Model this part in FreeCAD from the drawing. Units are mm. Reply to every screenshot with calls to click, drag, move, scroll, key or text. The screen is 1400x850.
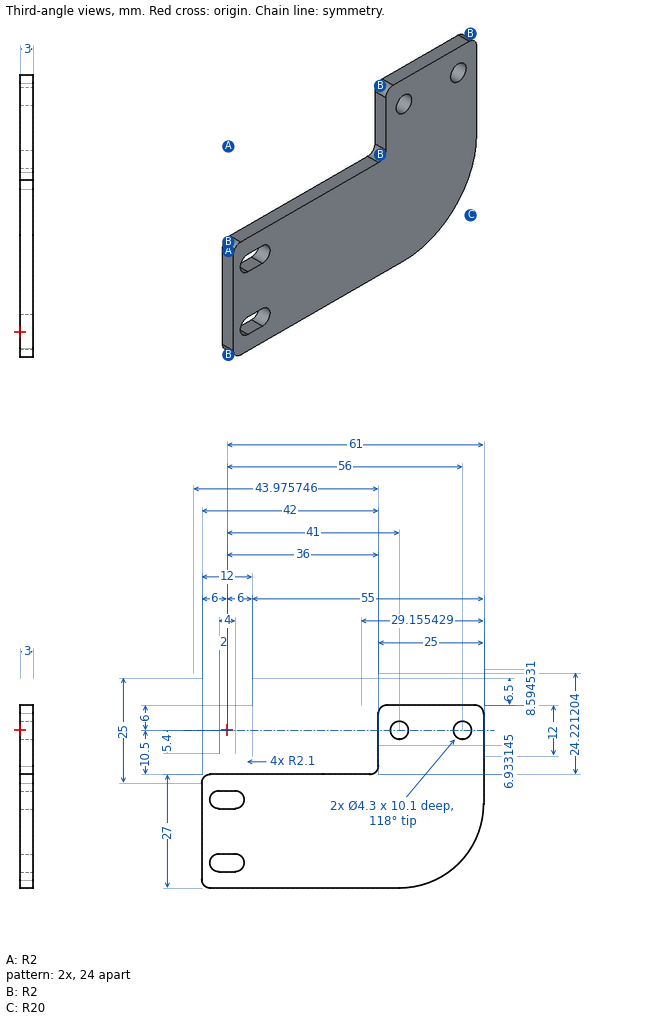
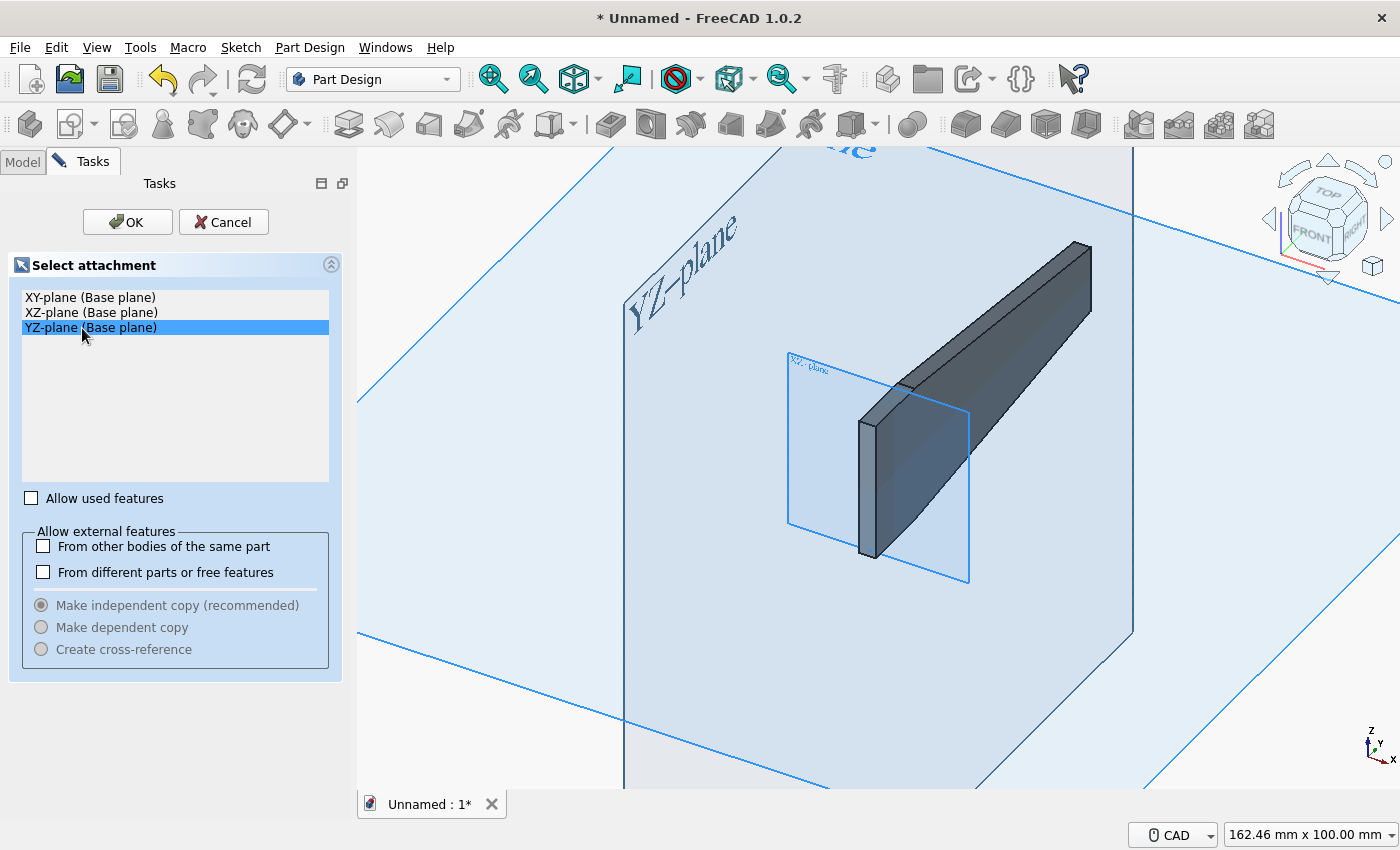
click(128, 222)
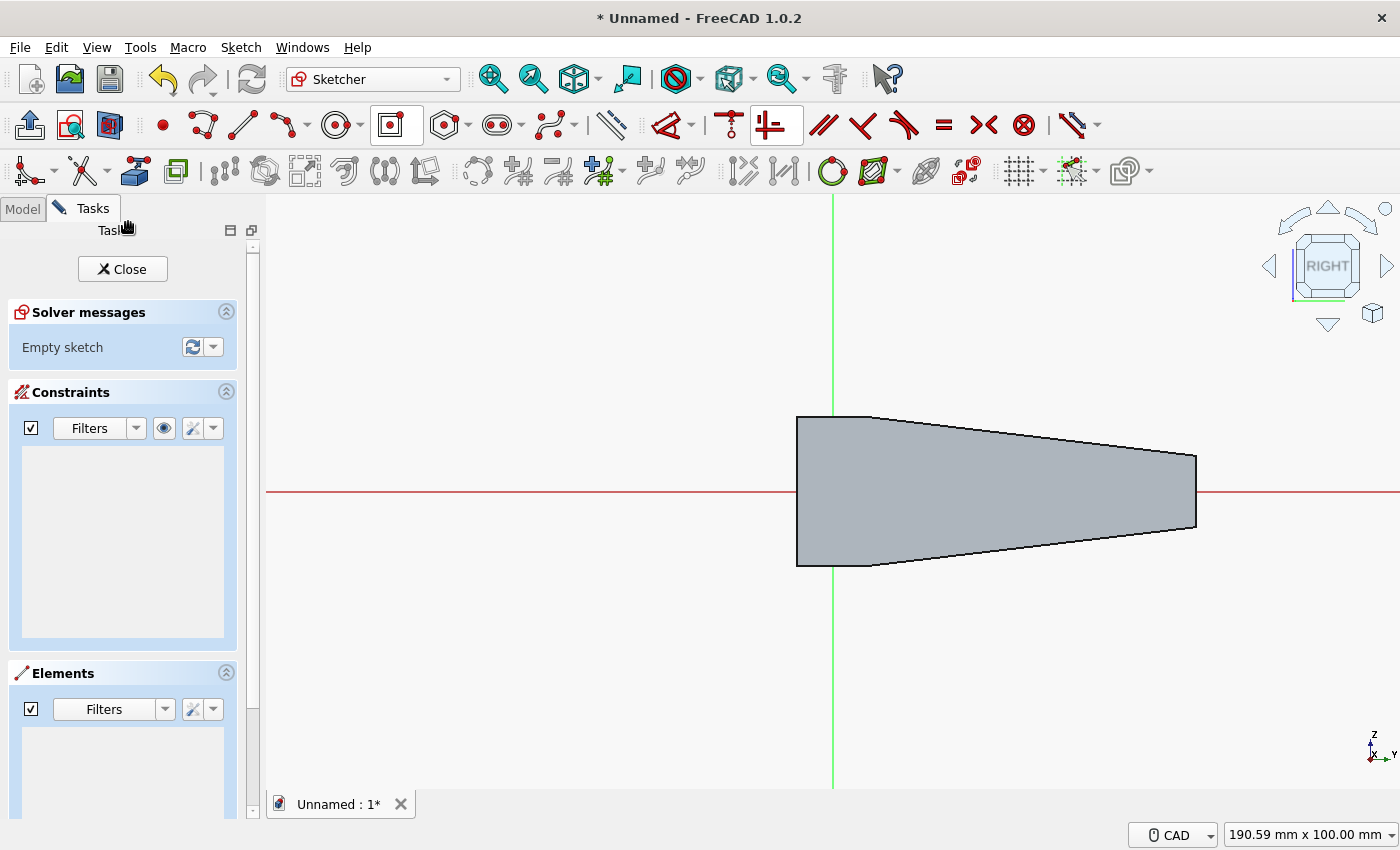
click(110, 126)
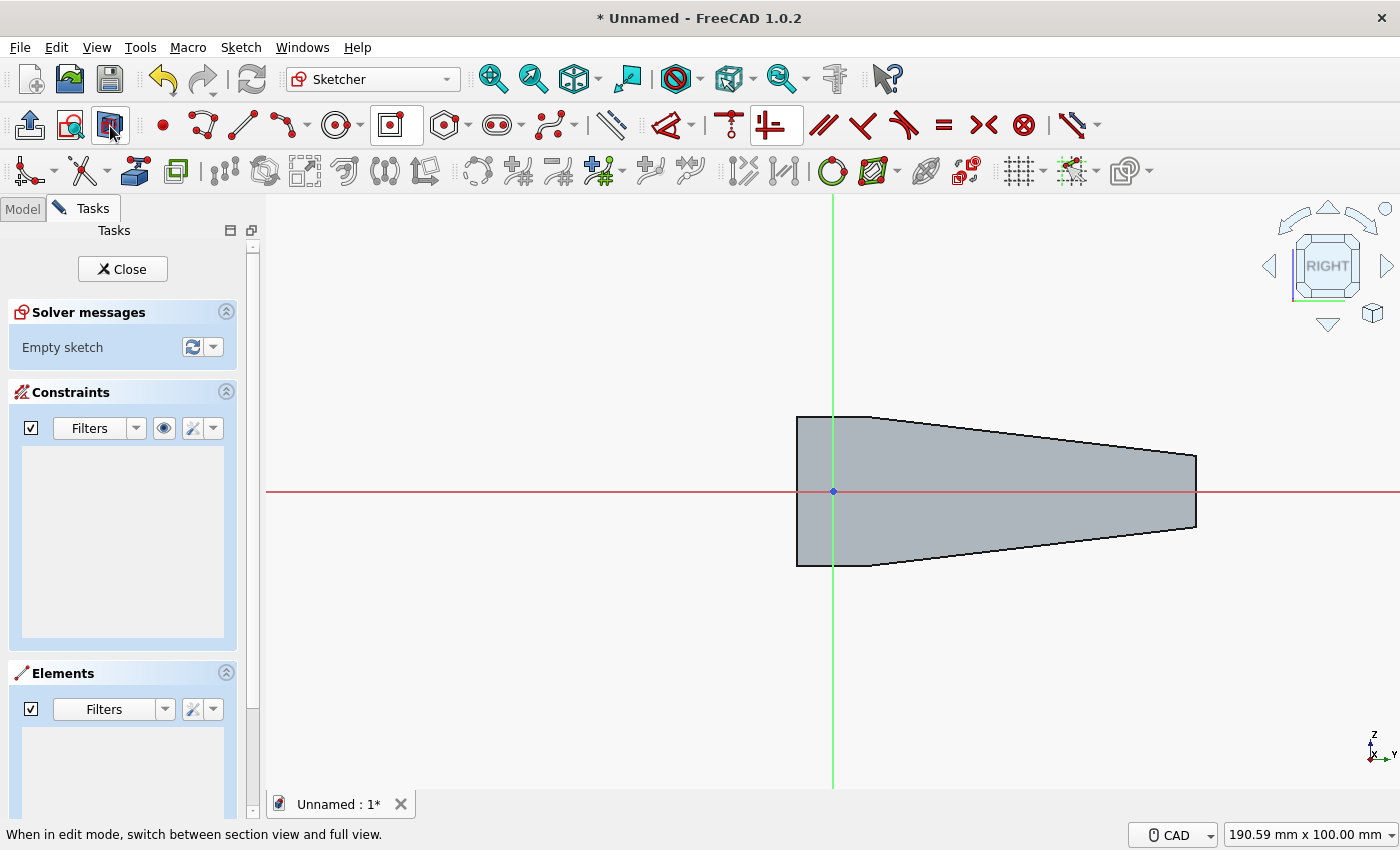
scroll(863, 492, up, 6)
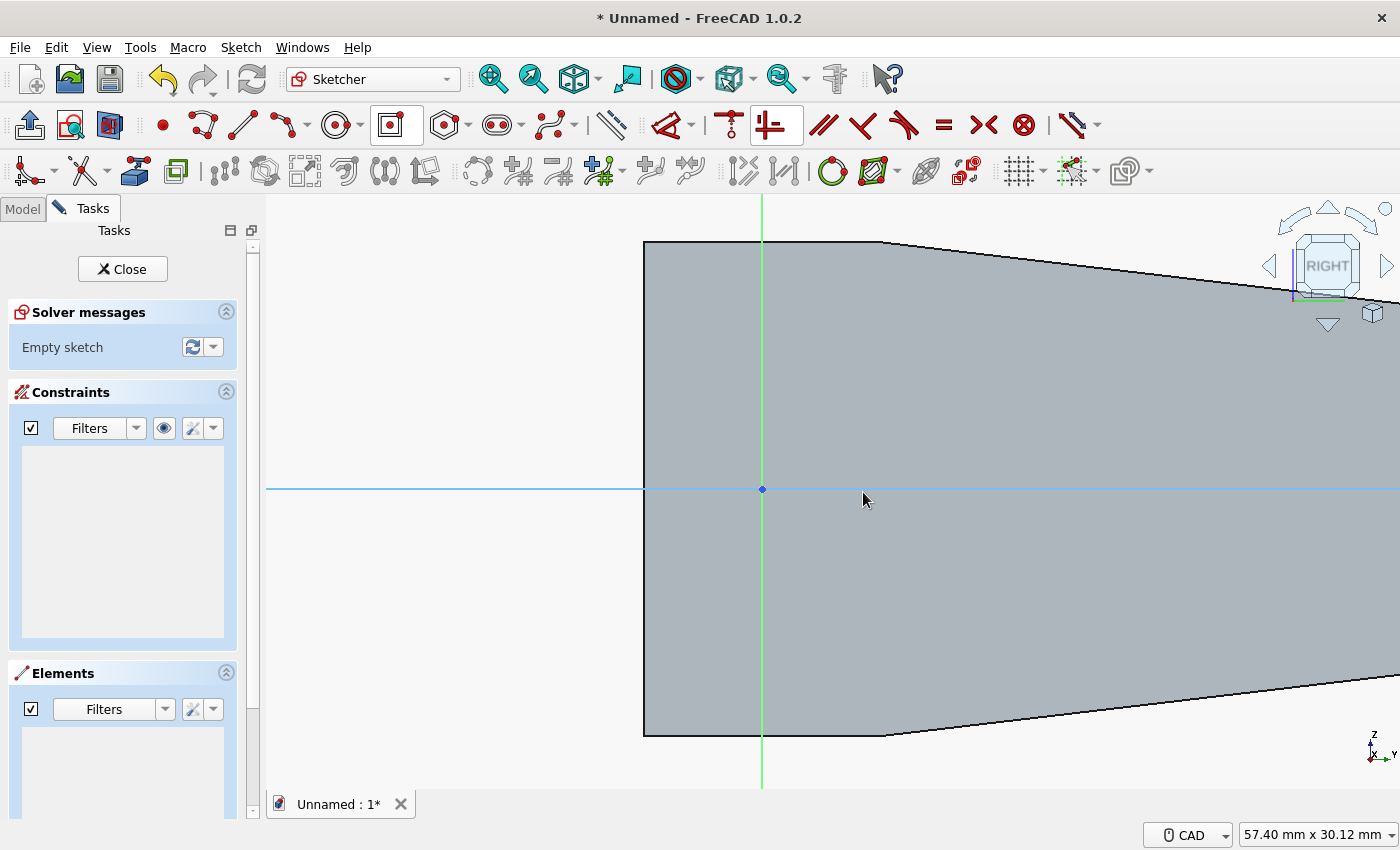
key(g)
key(s)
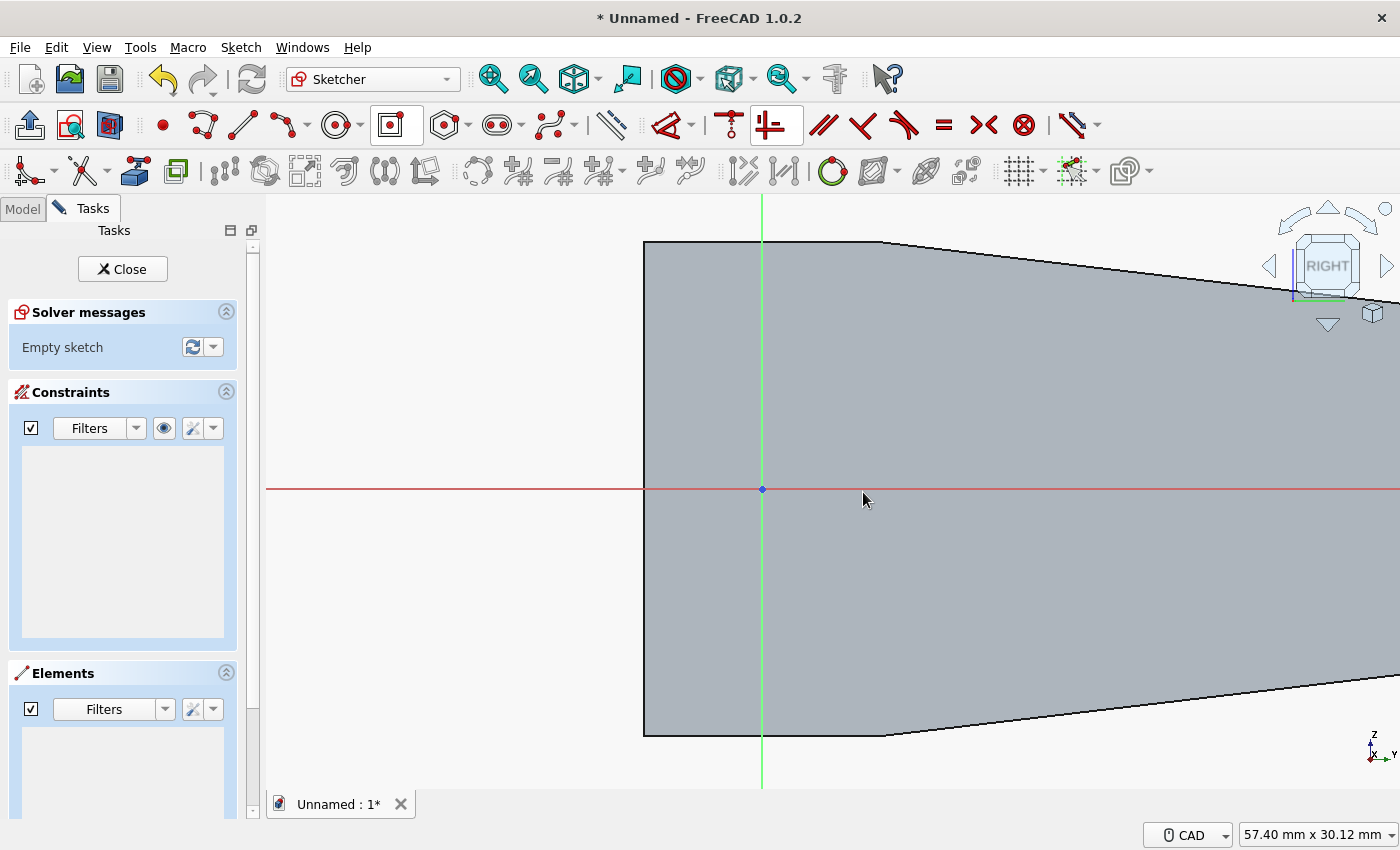
click(723, 637)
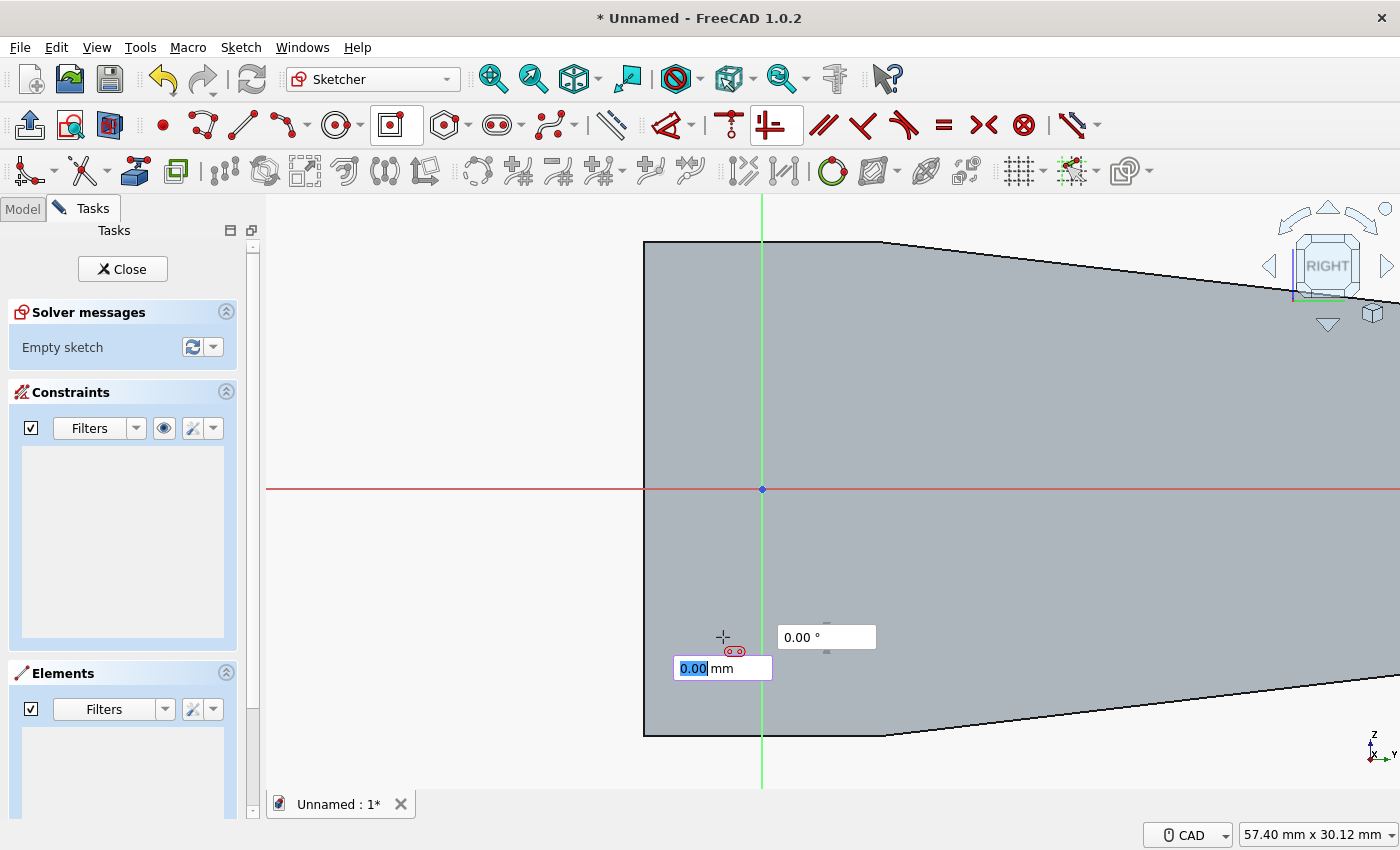
click(802, 637)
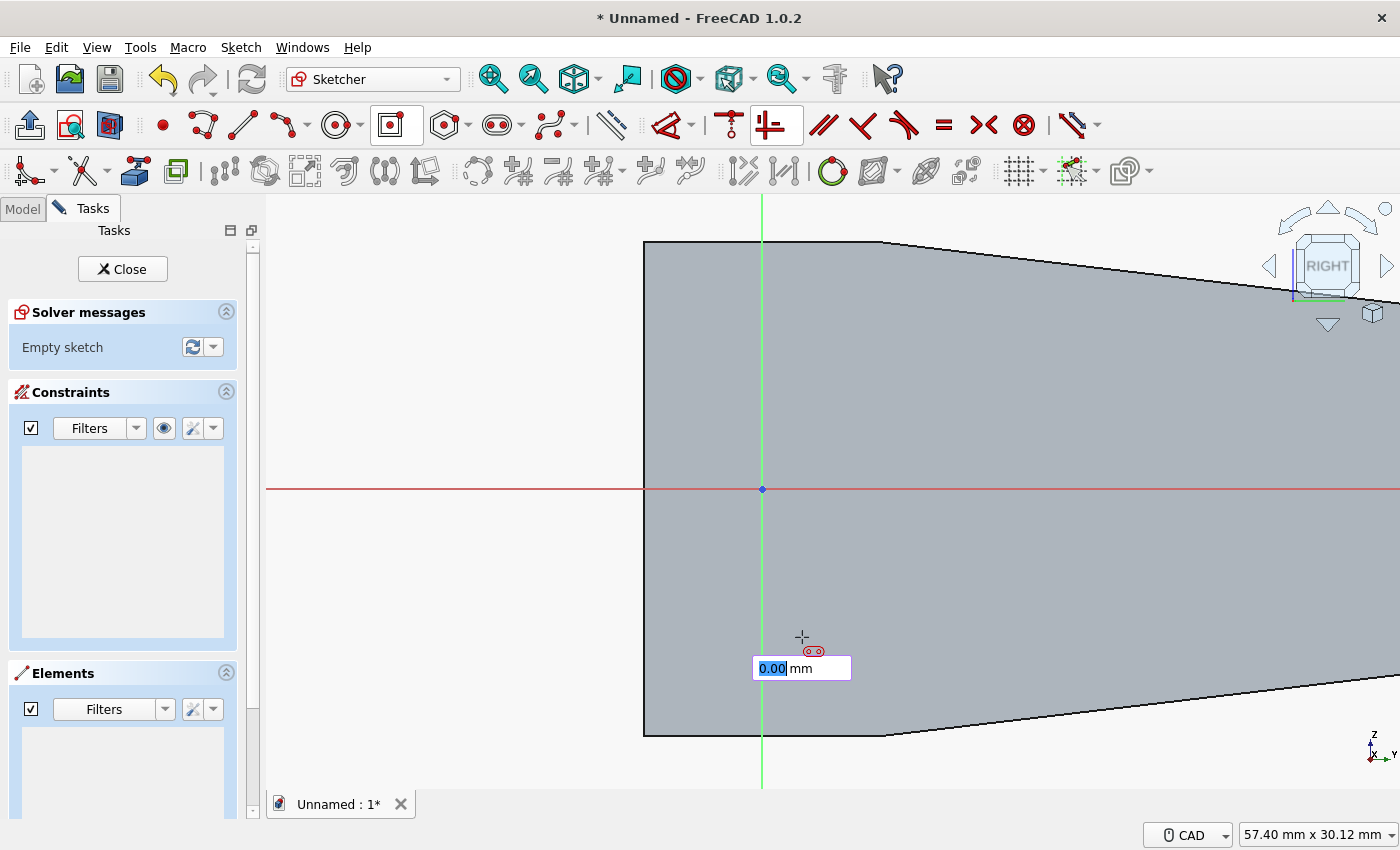
scroll(750, 596, up, 2)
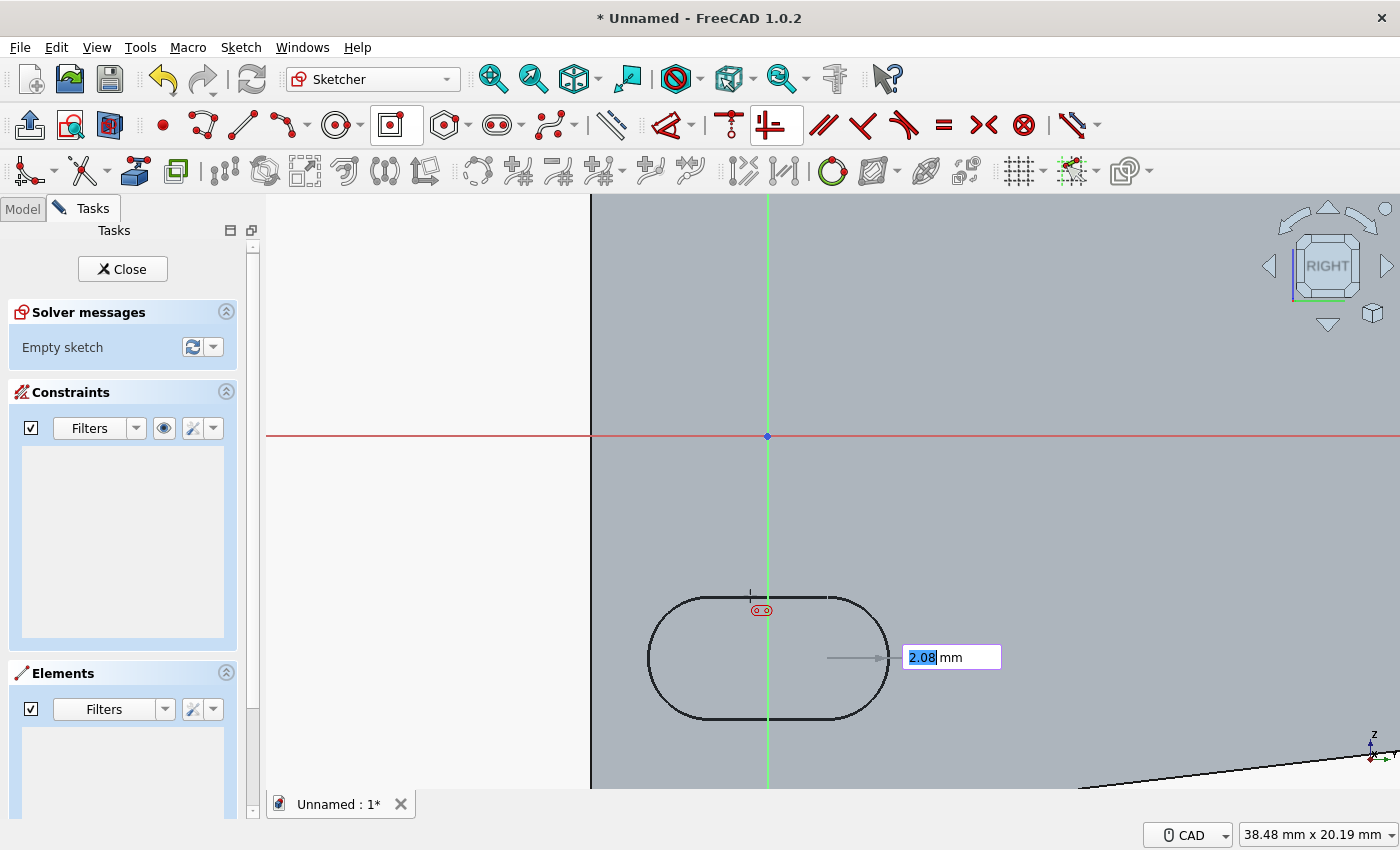
click(750, 595)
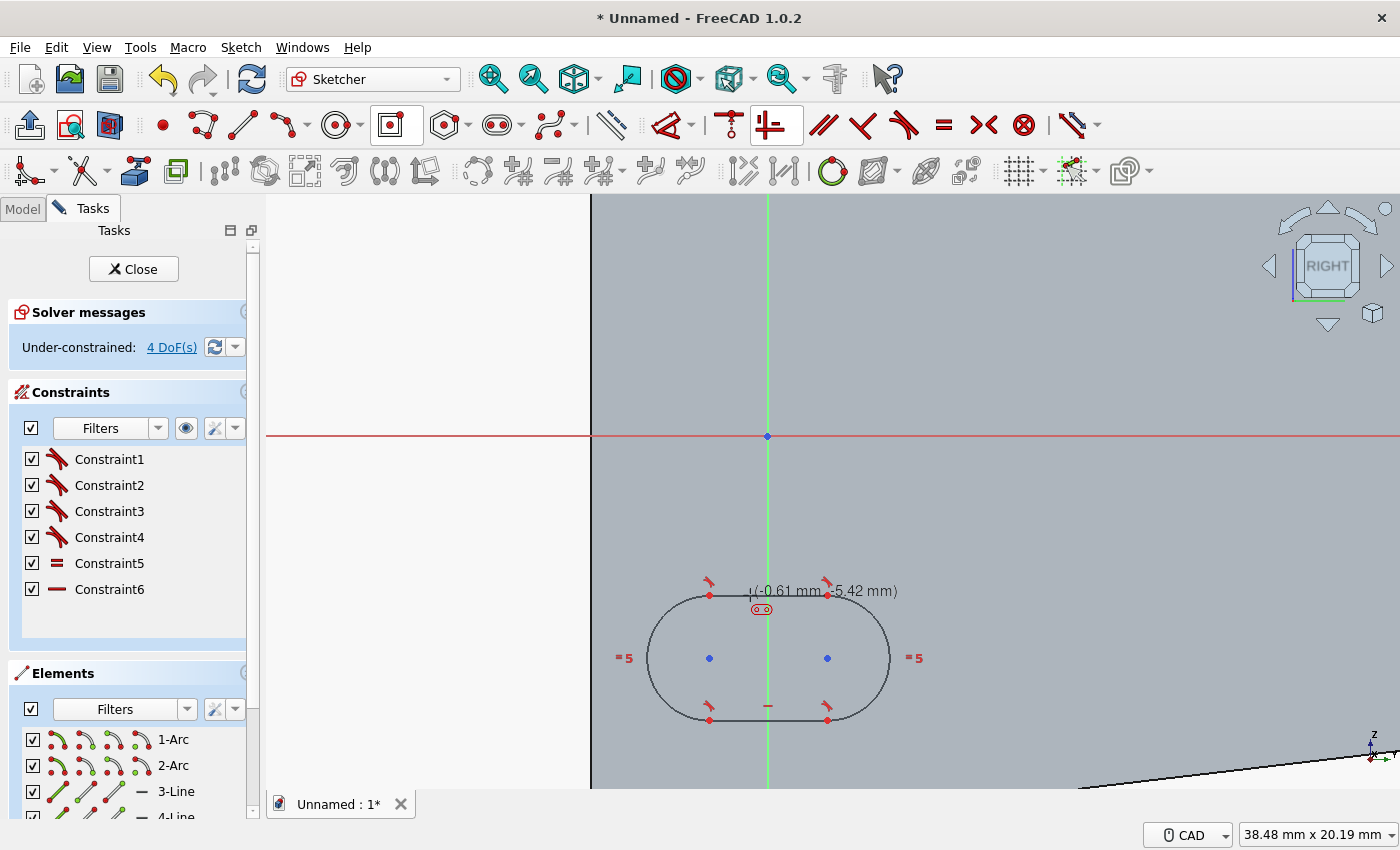
scroll(757, 604, down, 2)